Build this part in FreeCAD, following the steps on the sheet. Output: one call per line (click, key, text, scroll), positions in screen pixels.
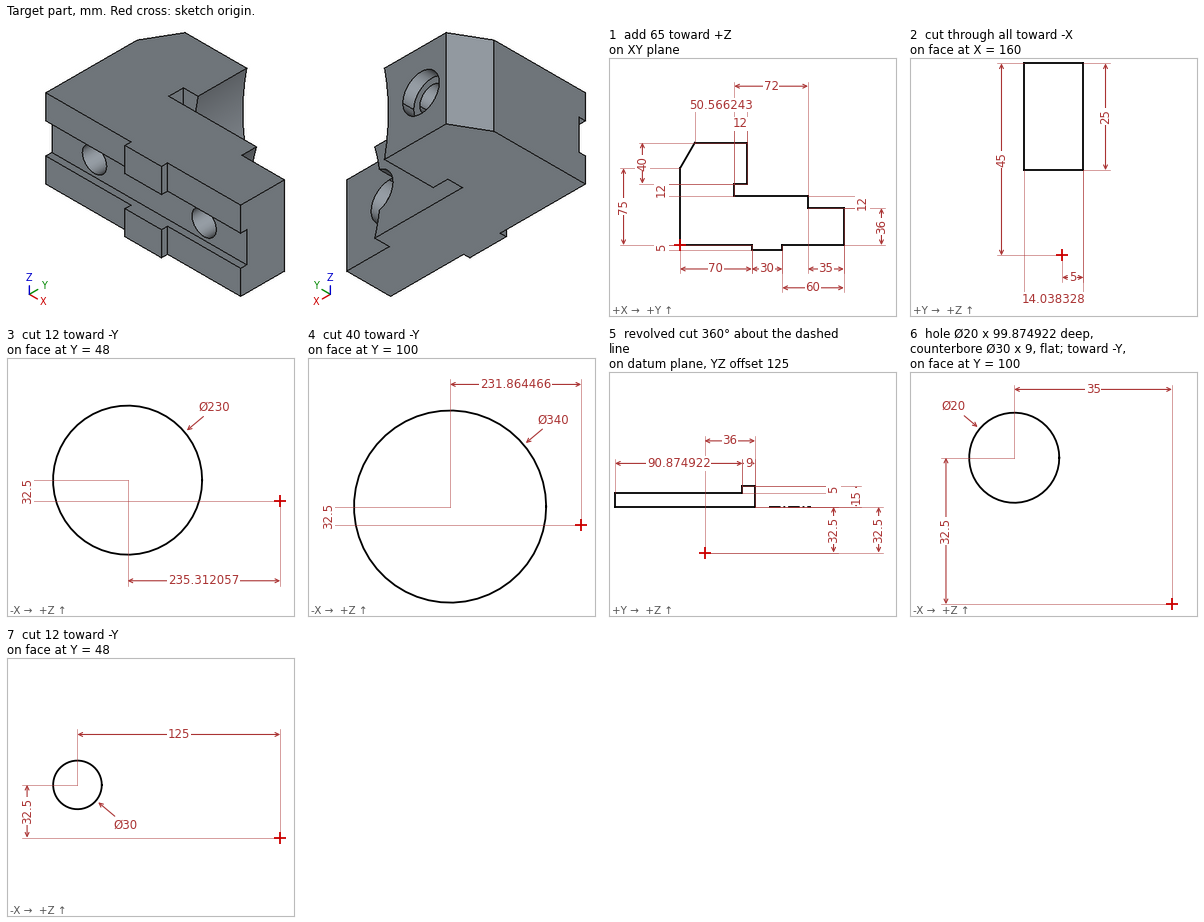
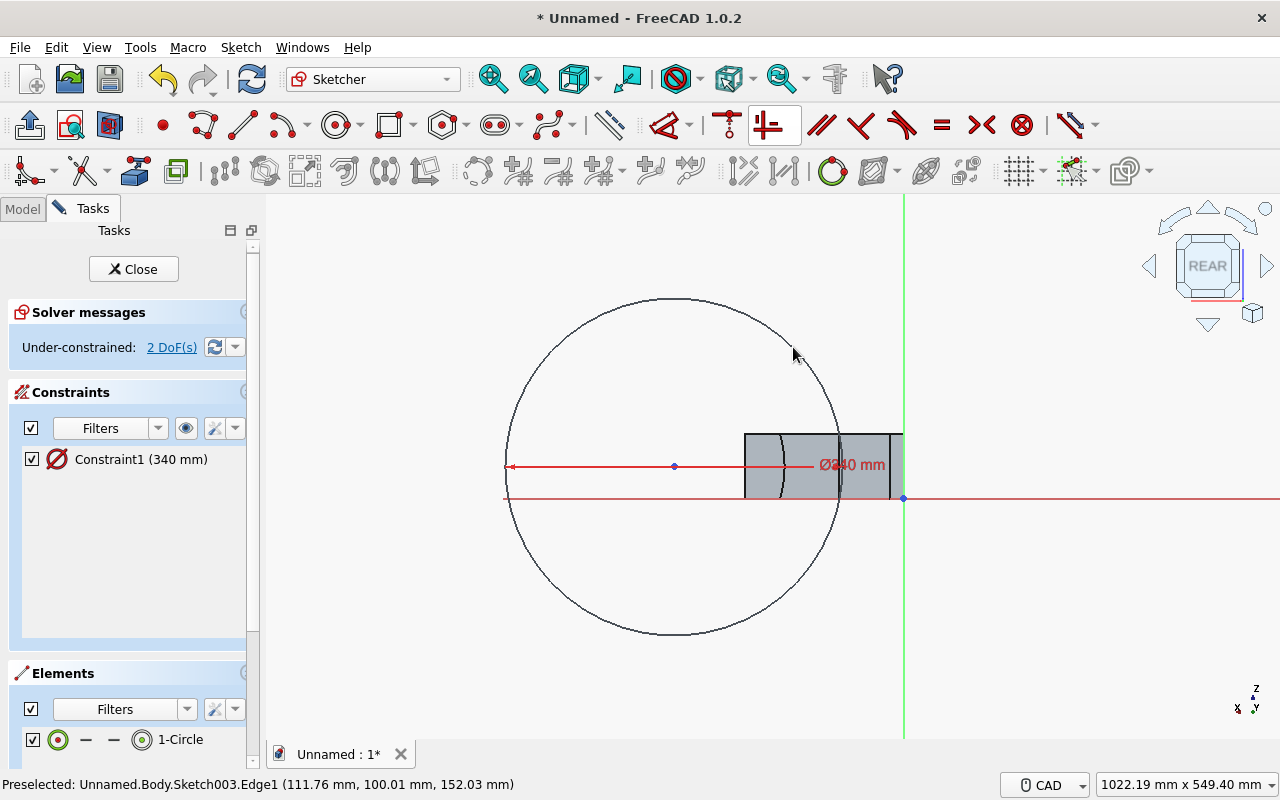
click(664, 126)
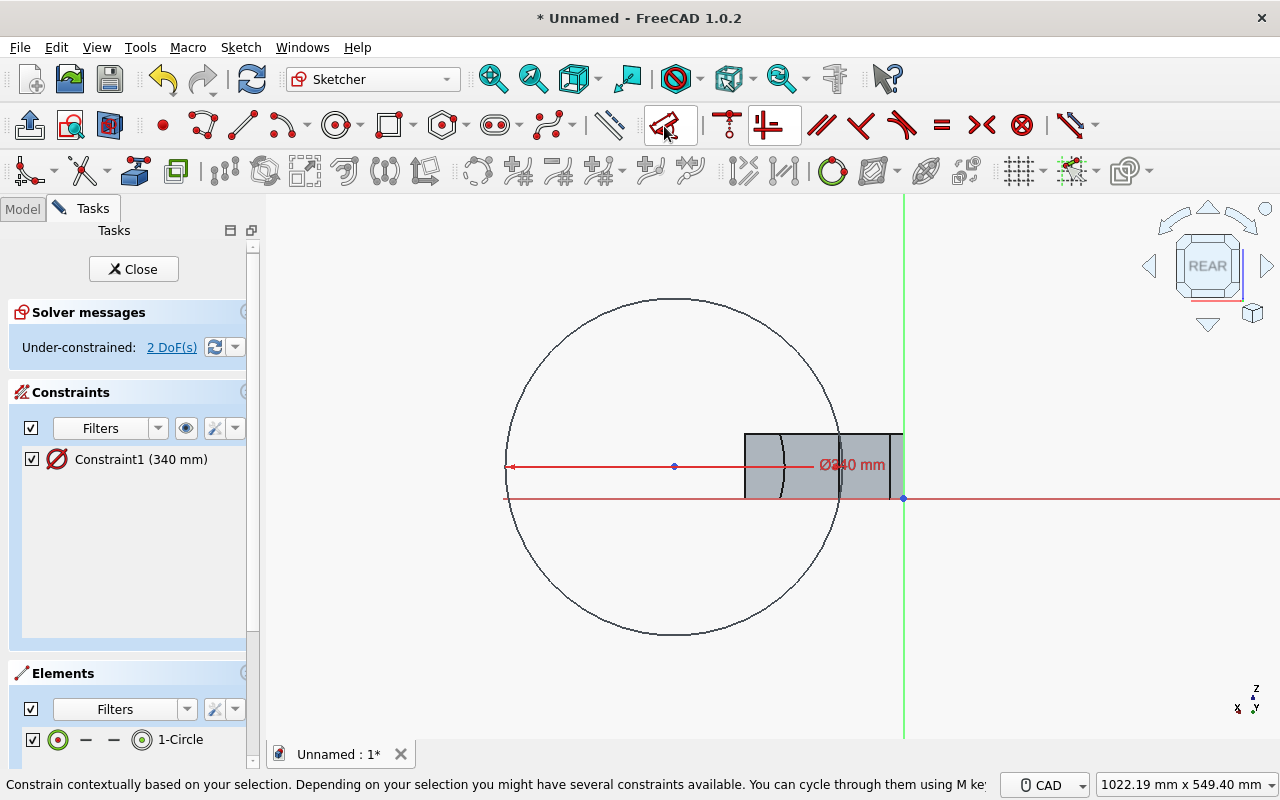
scroll(674, 467, up, 2)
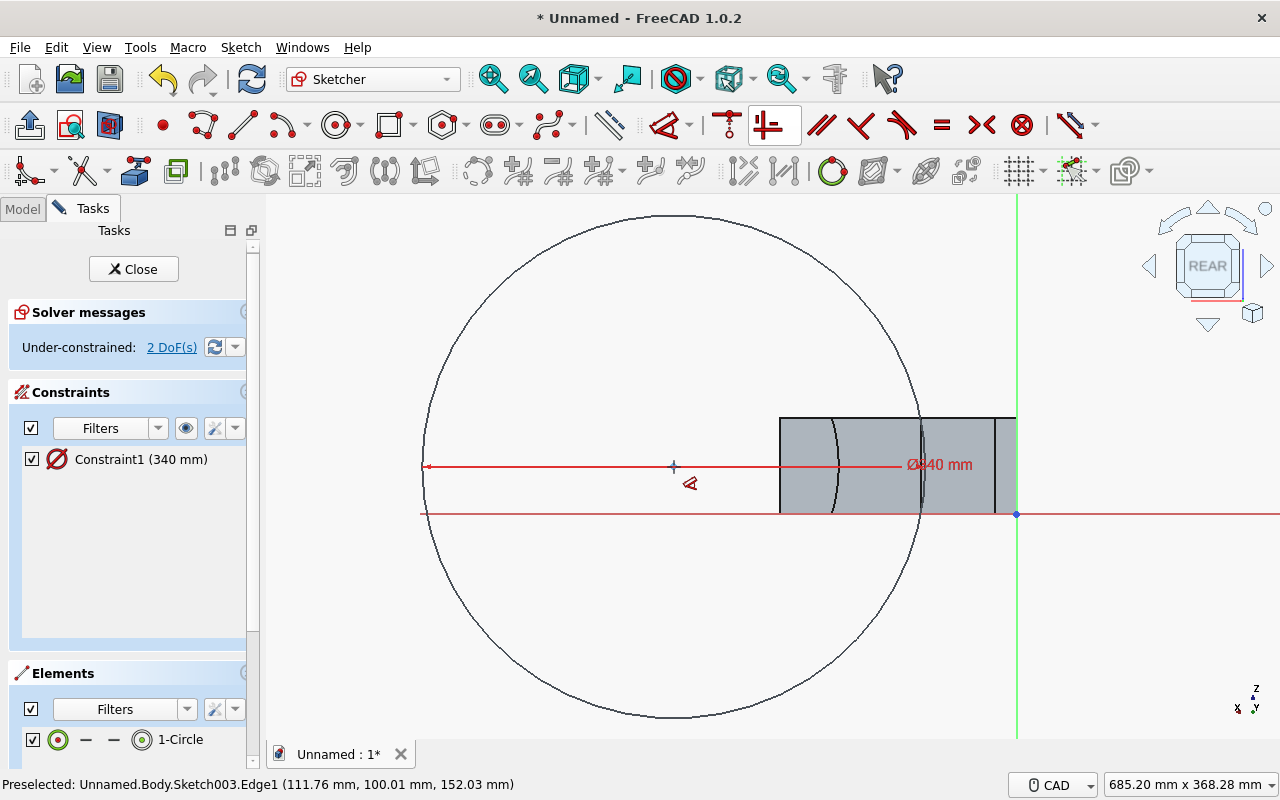
click(674, 467)
click(1051, 490)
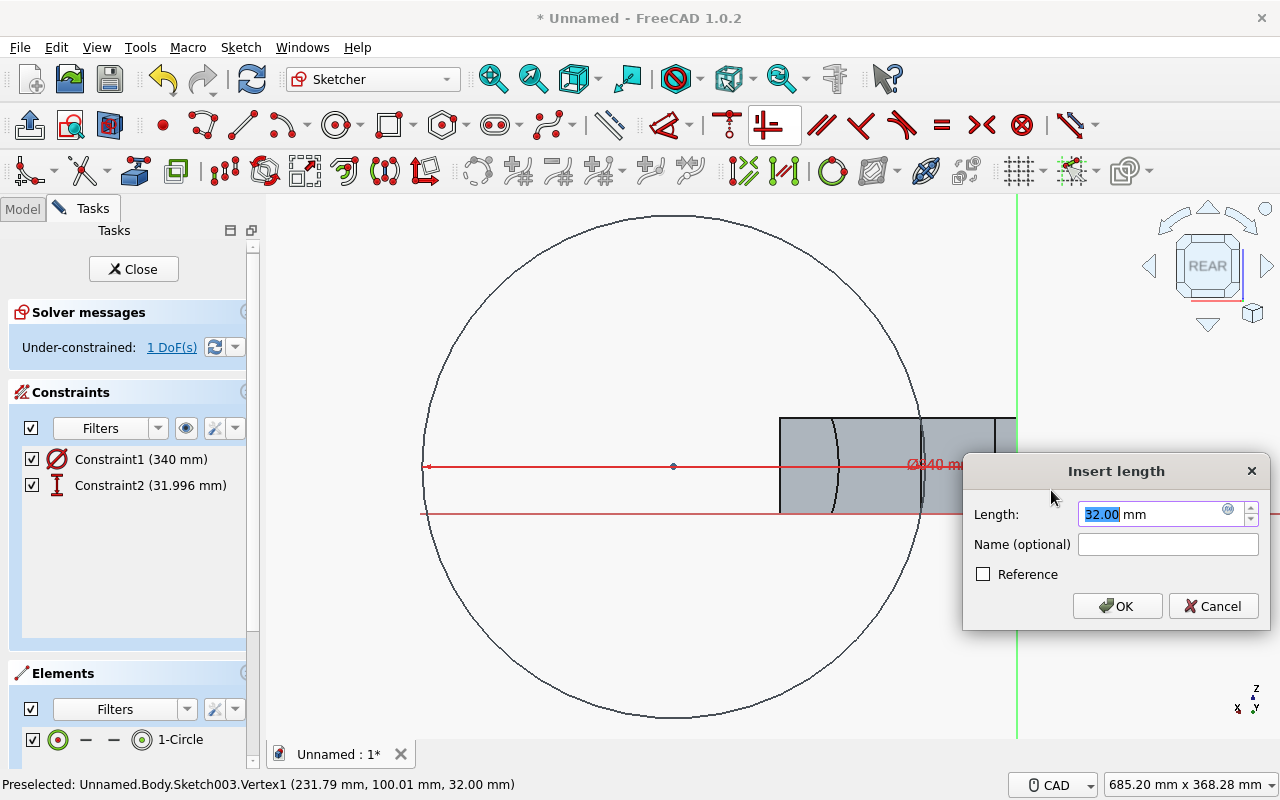
text(32.5)
key(Return)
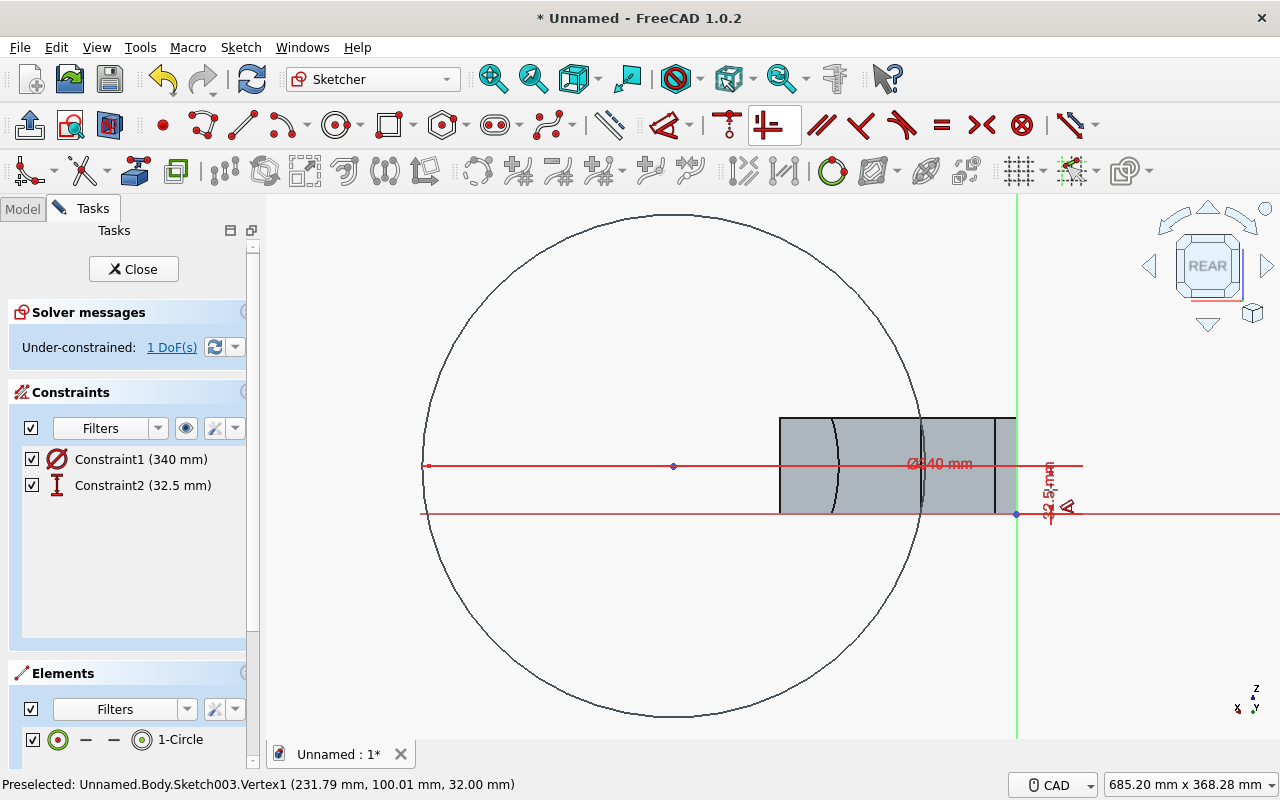
click(674, 466)
click(845, 548)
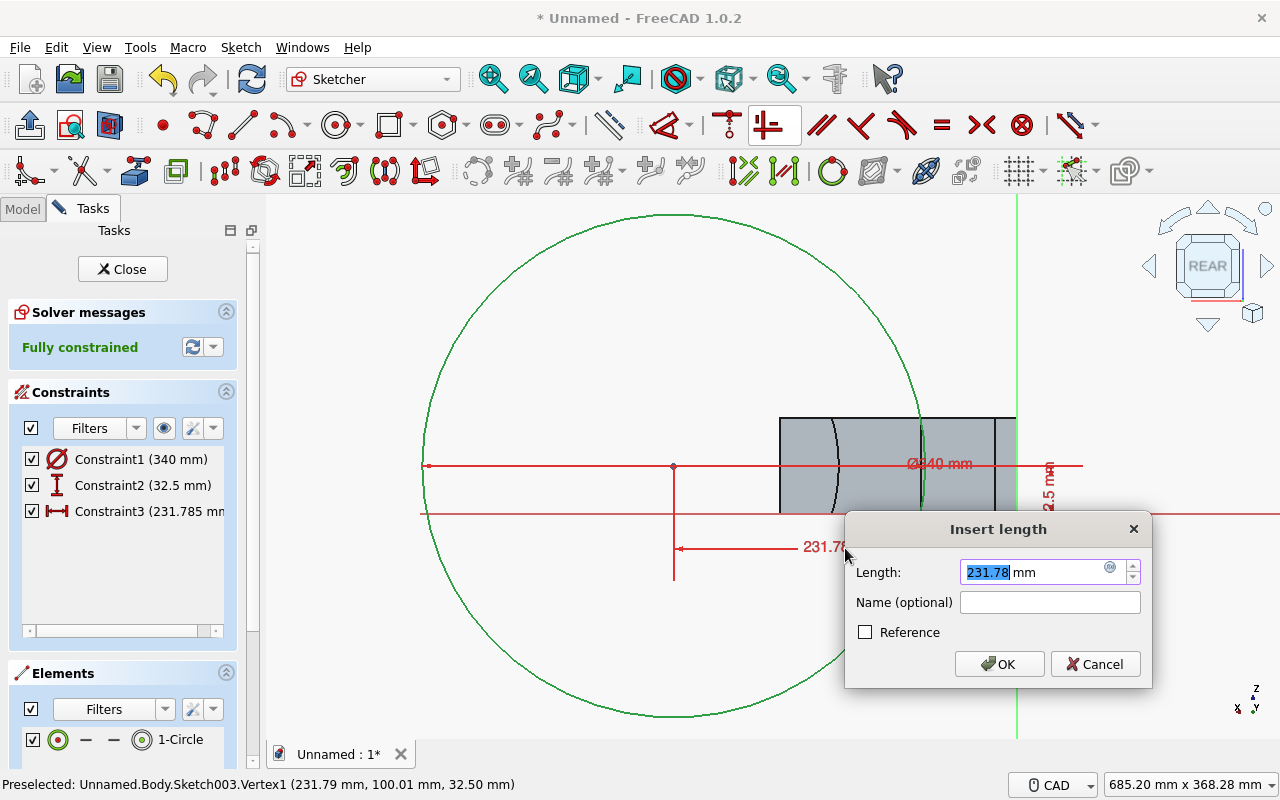
text(231.864466)
key(Return)
key(Escape)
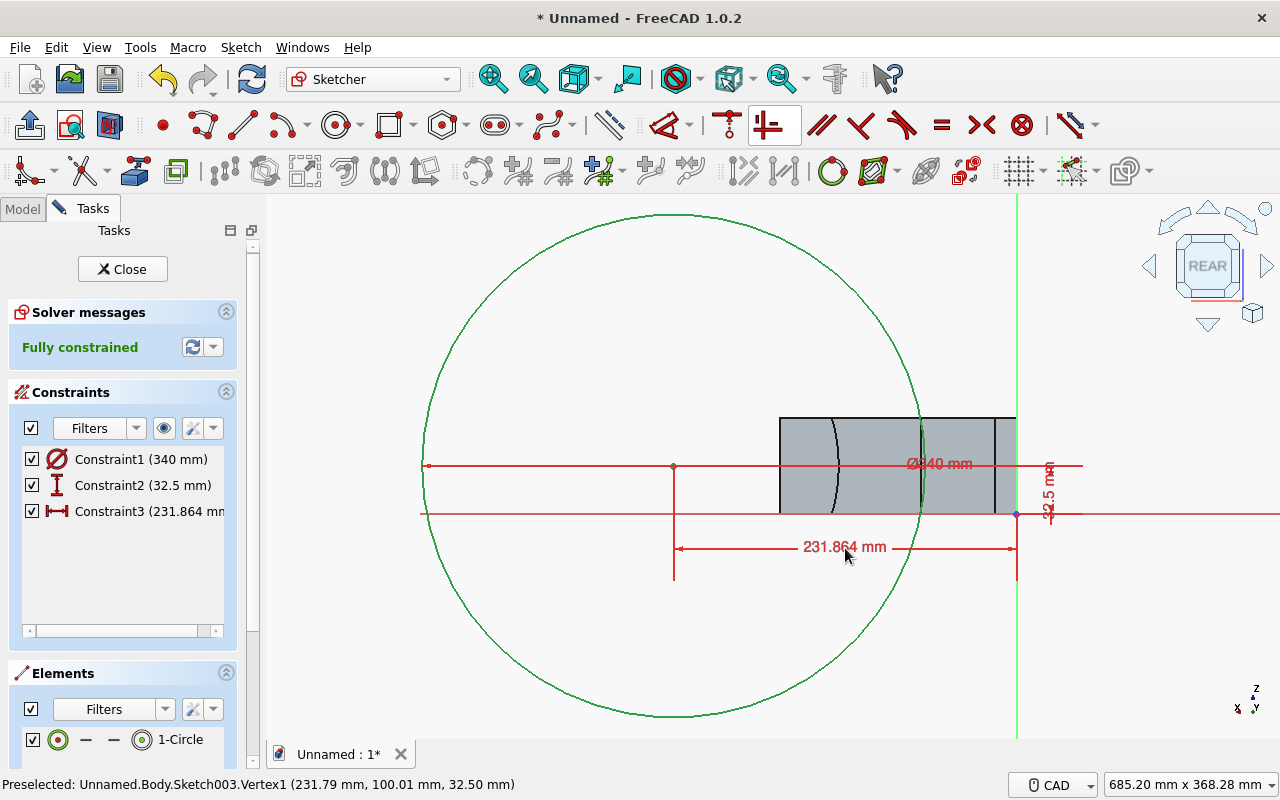
click(123, 269)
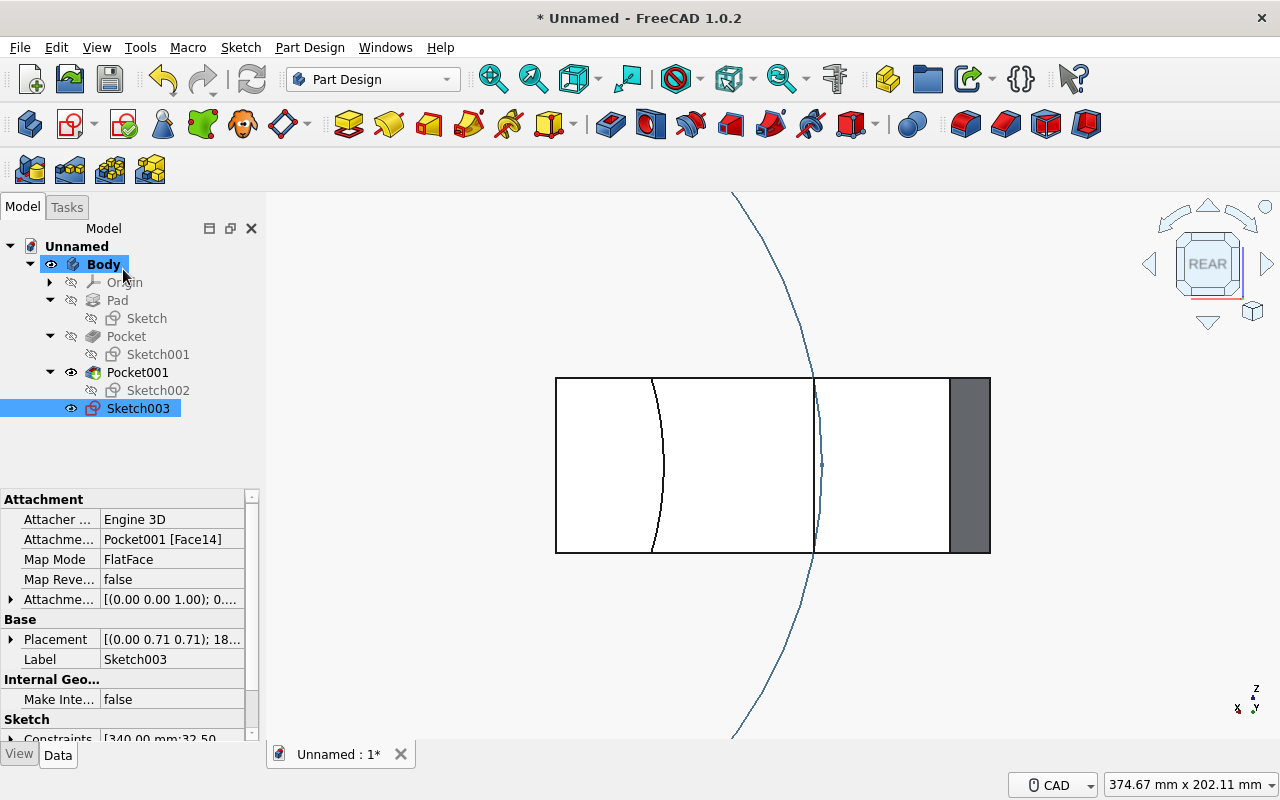
click(612, 124)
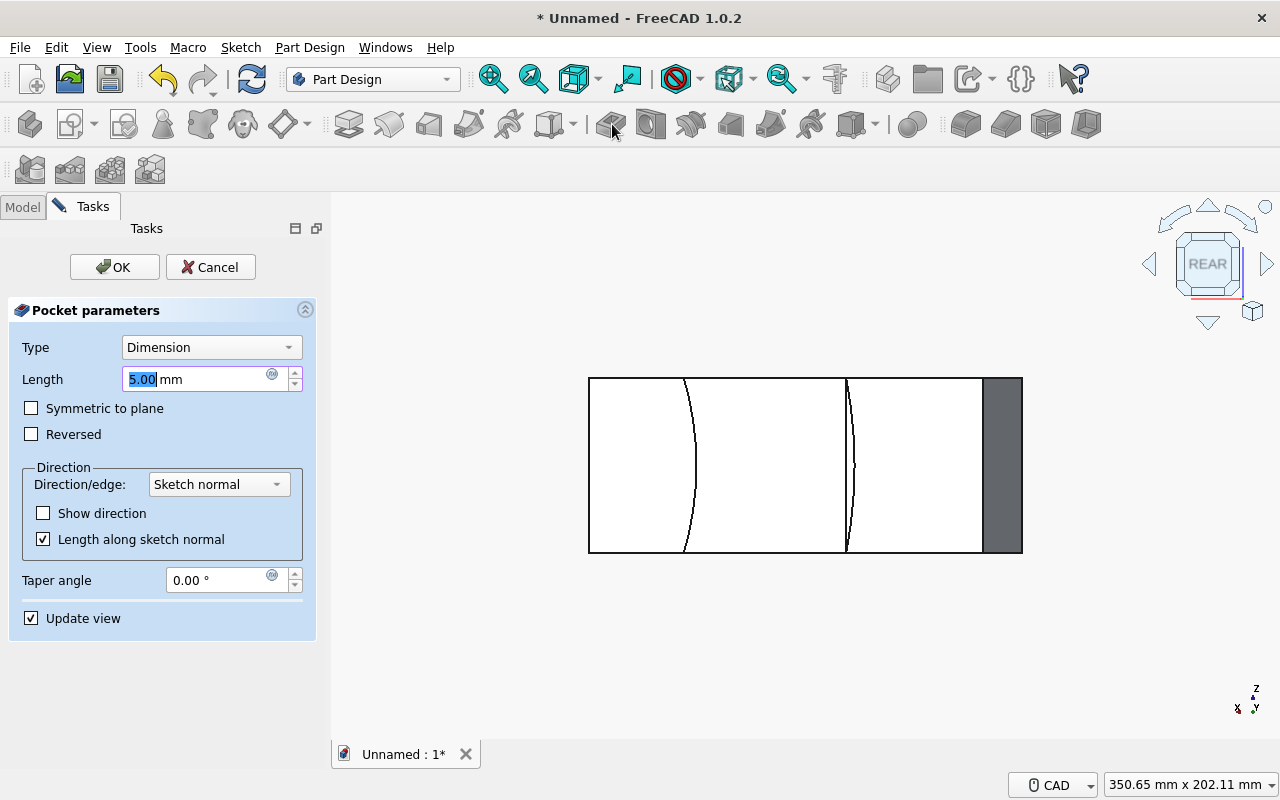
text(40)
key(Tab)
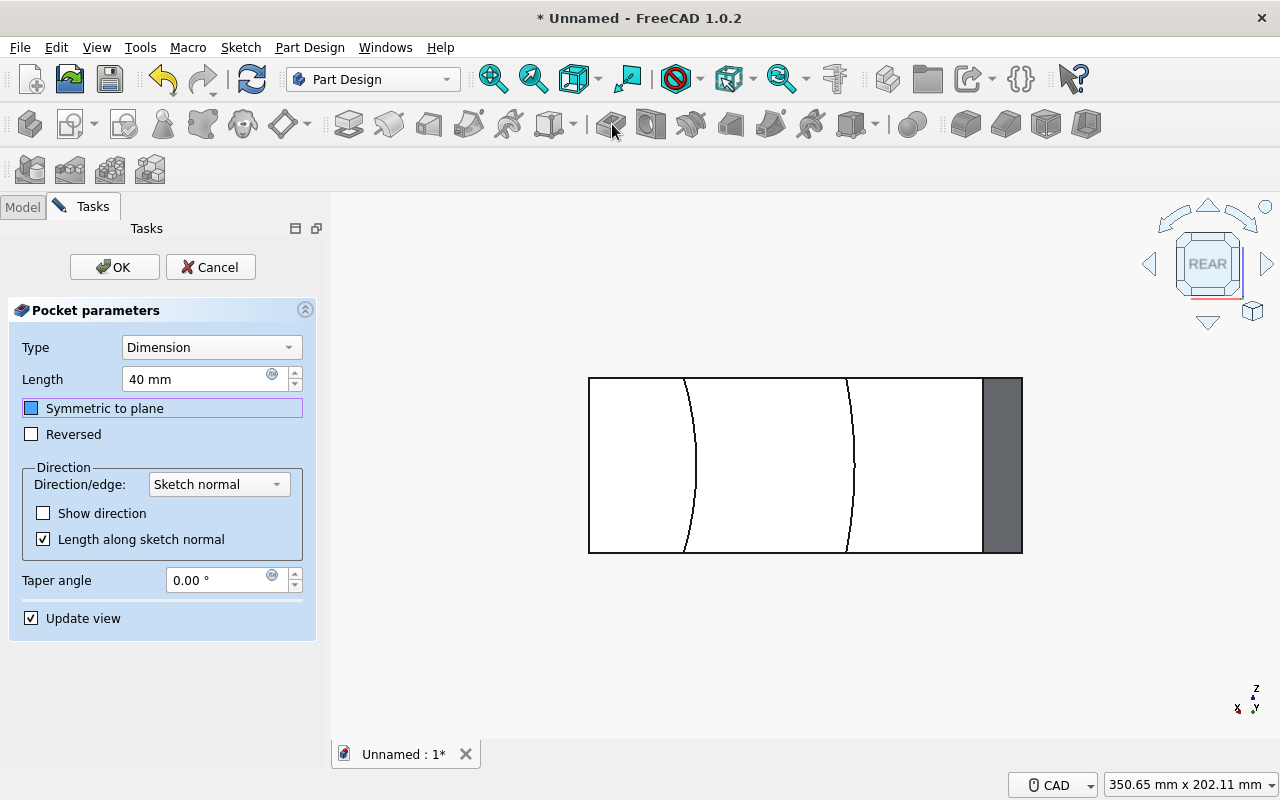
click(115, 267)